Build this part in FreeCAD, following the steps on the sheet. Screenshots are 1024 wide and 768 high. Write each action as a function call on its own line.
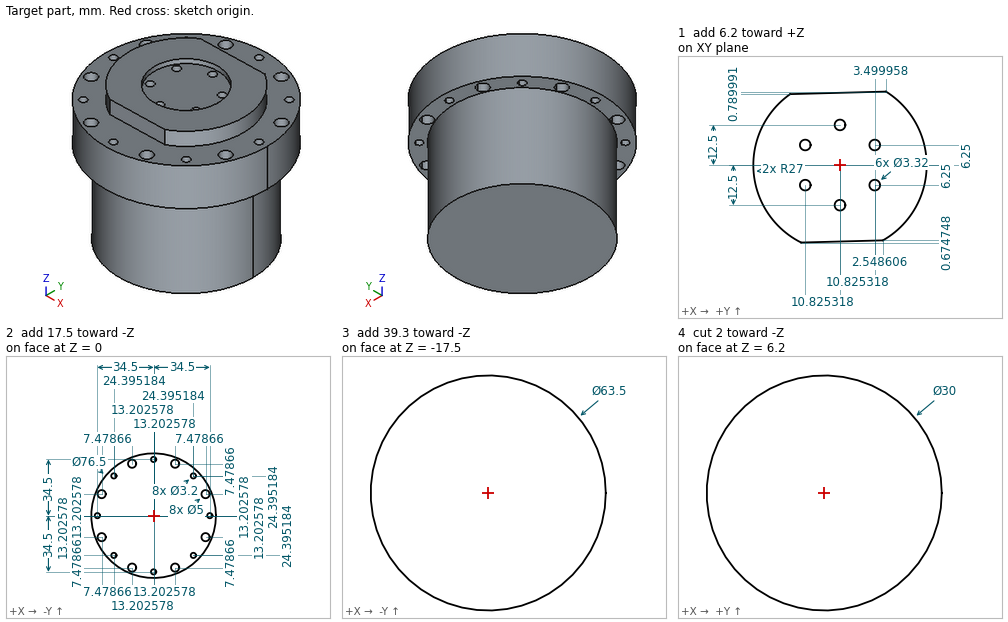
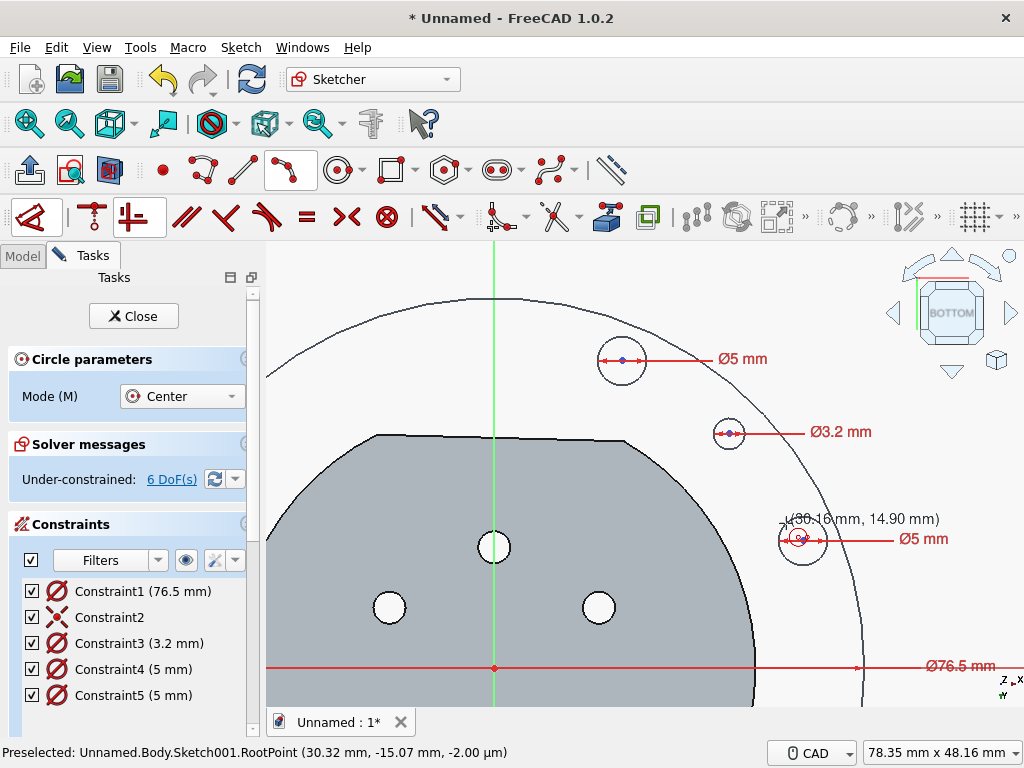
scroll(494, 334, up, 2)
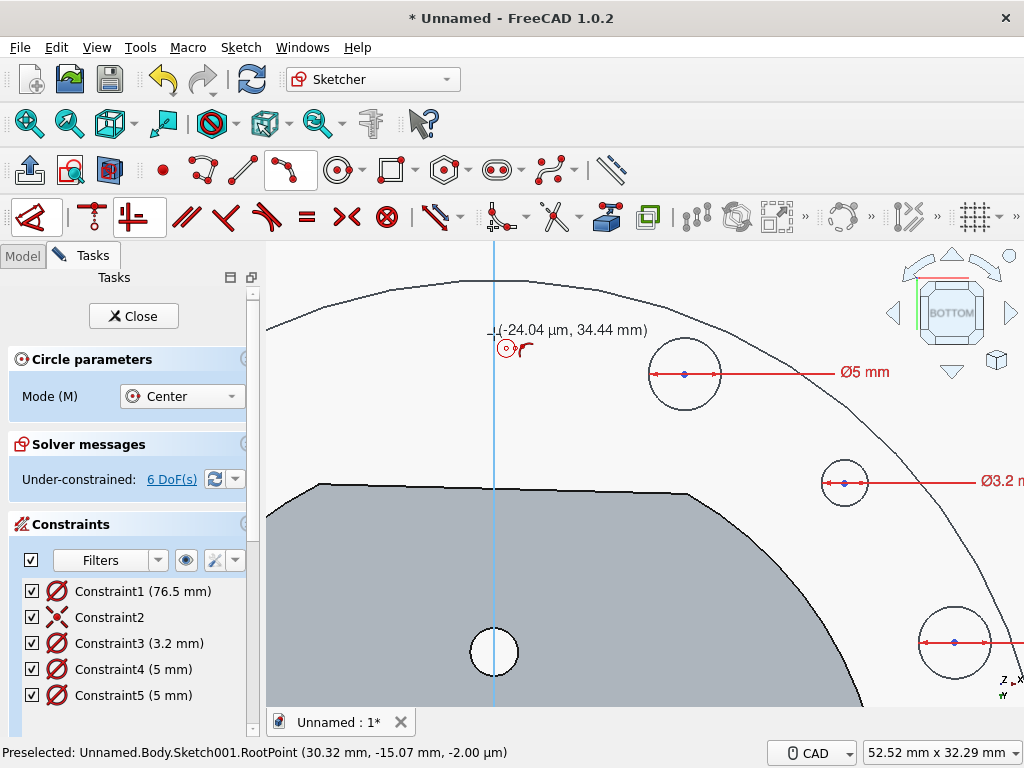
scroll(603, 357, down, 7)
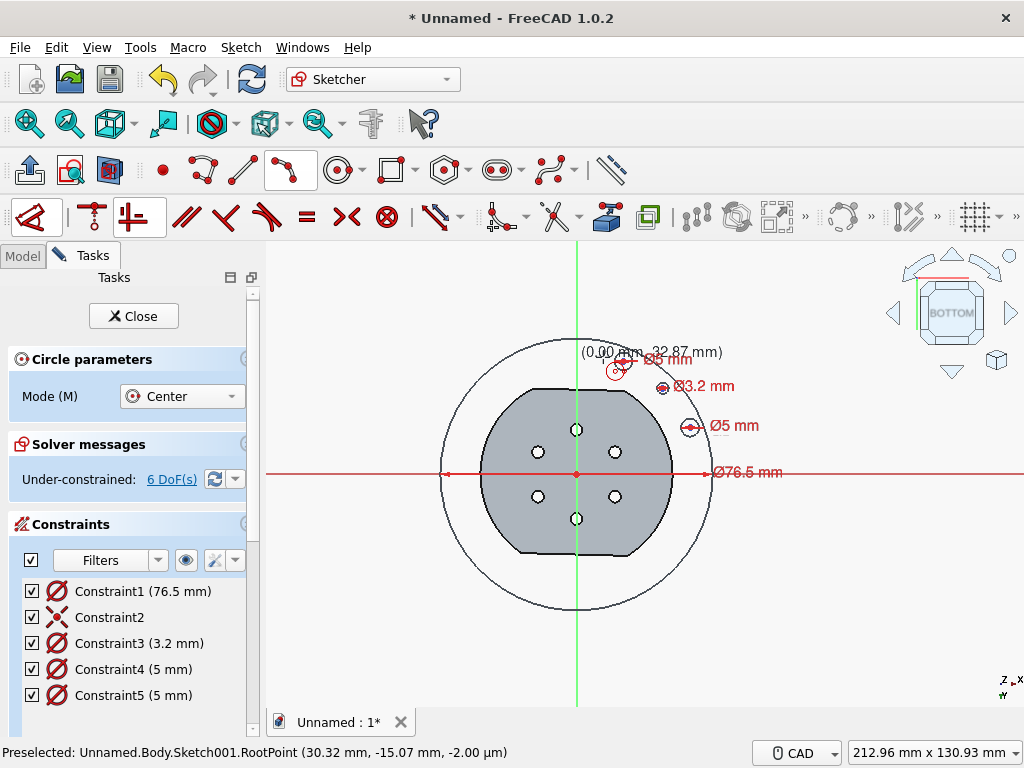
click(577, 352)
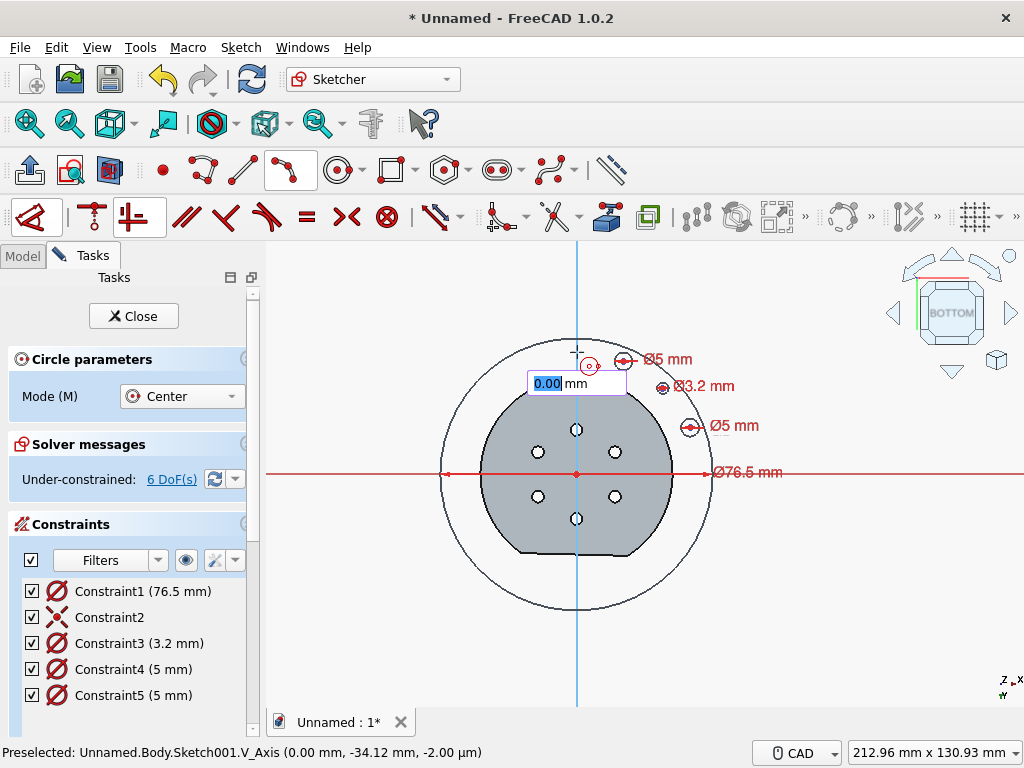
scroll(582, 350, up, 6)
move(581, 348)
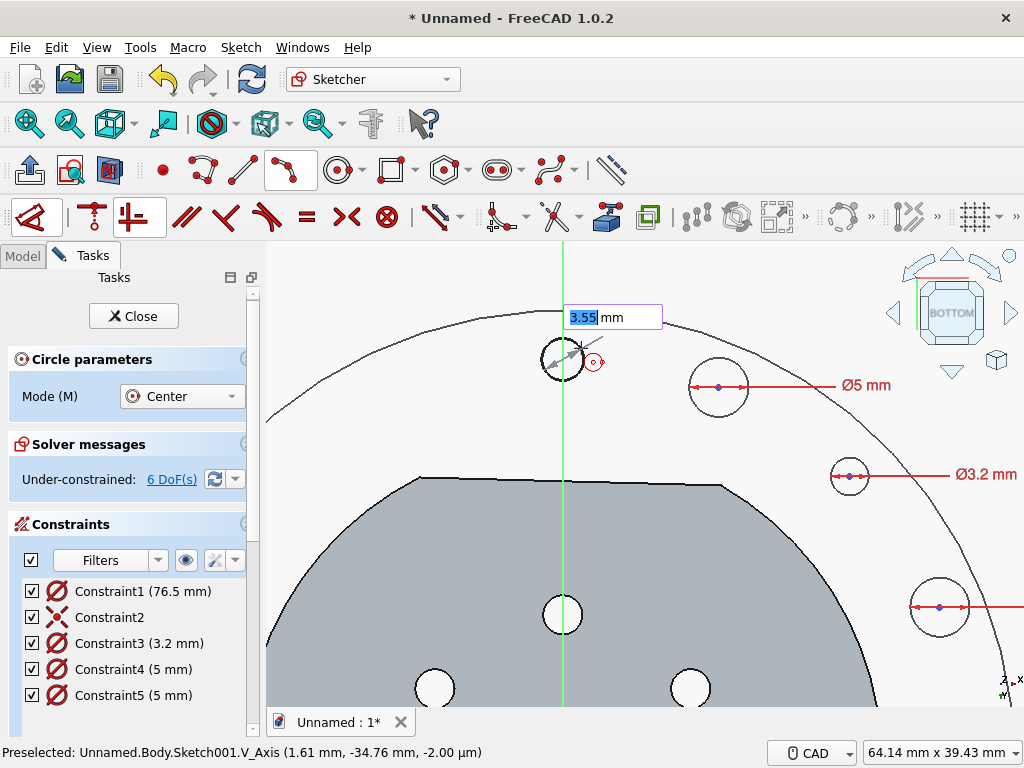
text(3.2)
key(Return)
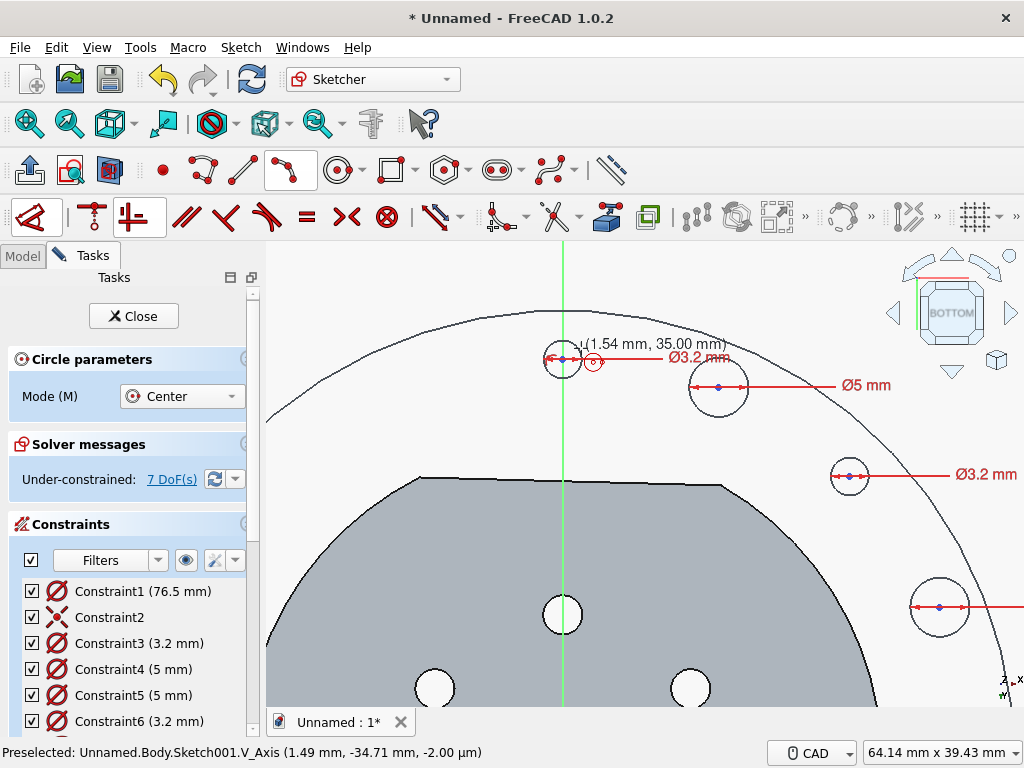
click(407, 386)
move(428, 365)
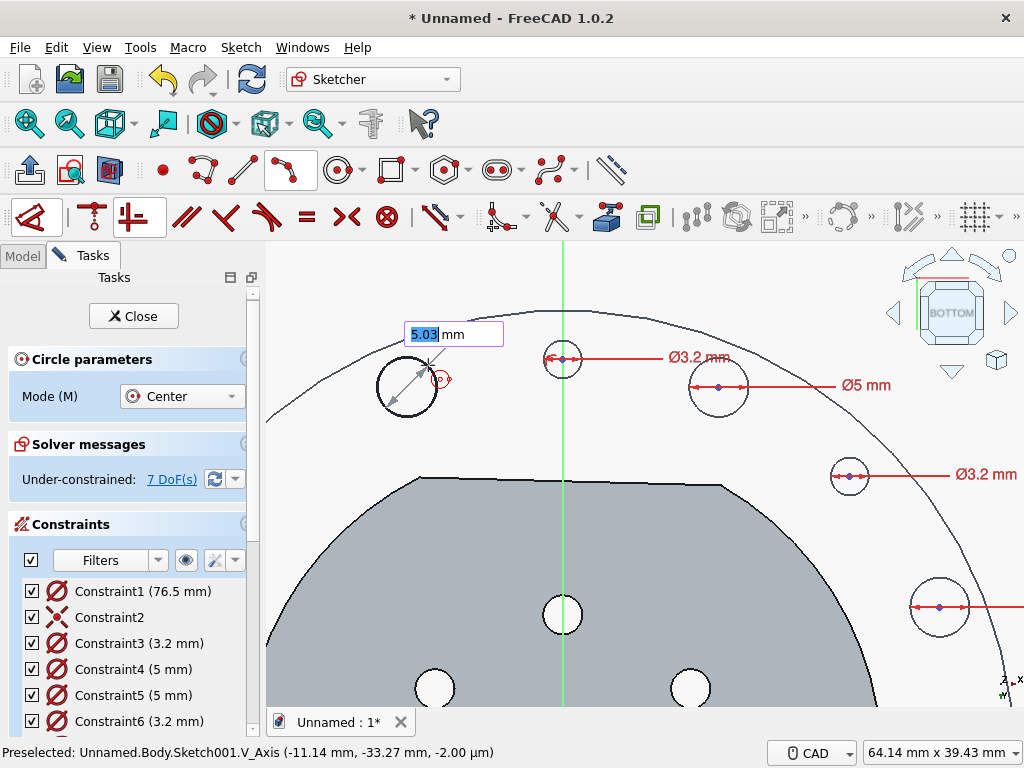
text(5)
key(Return)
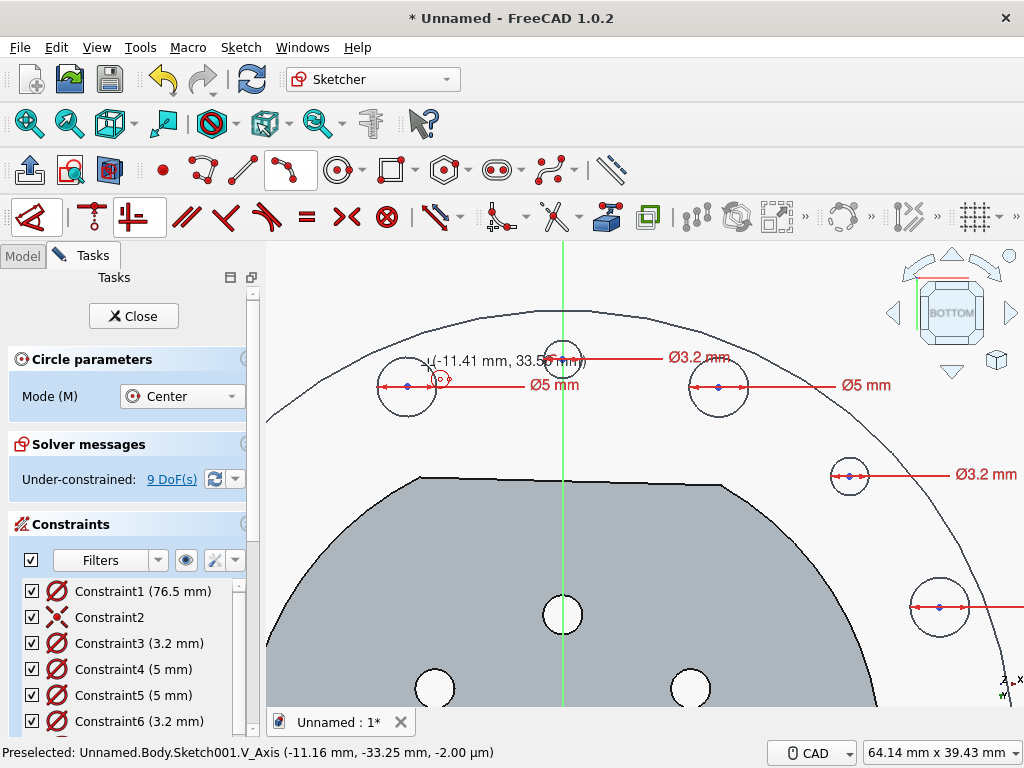
scroll(582, 350, down, 6)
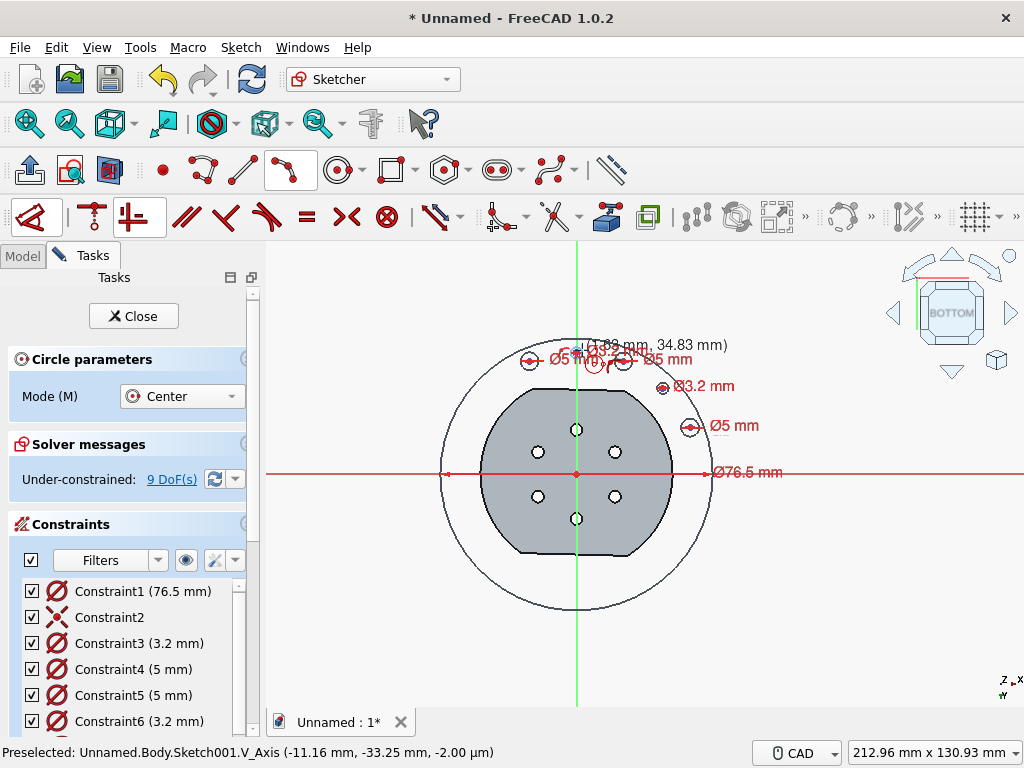
scroll(490, 388, up, 7)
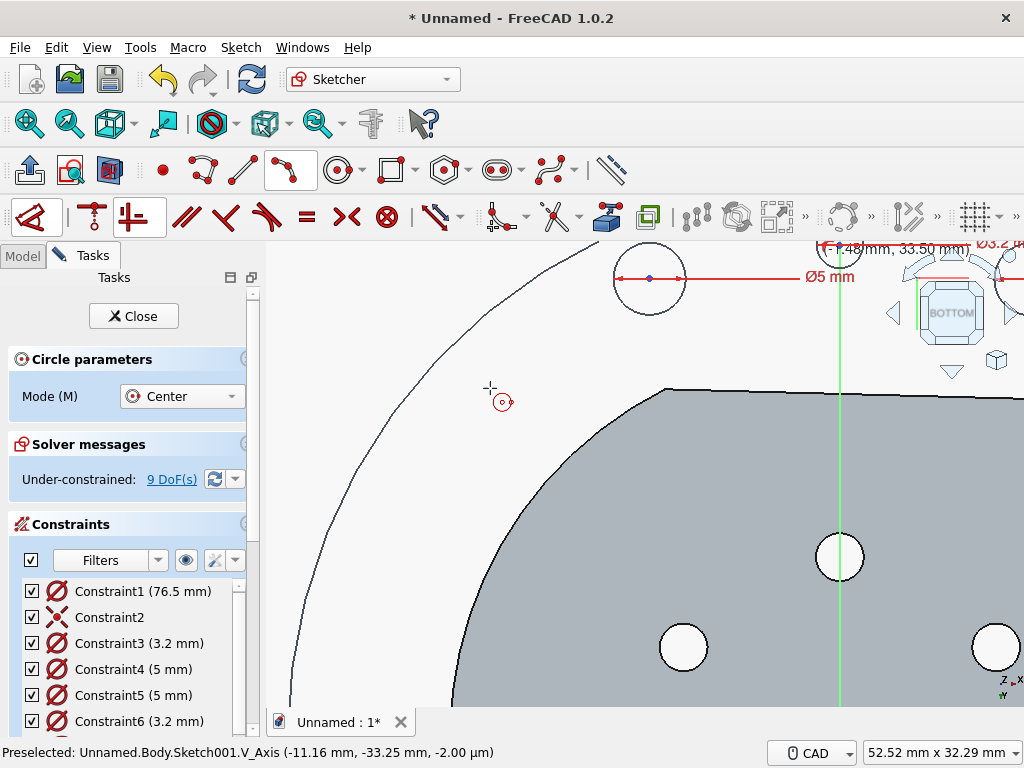
scroll(490, 388, down, 7)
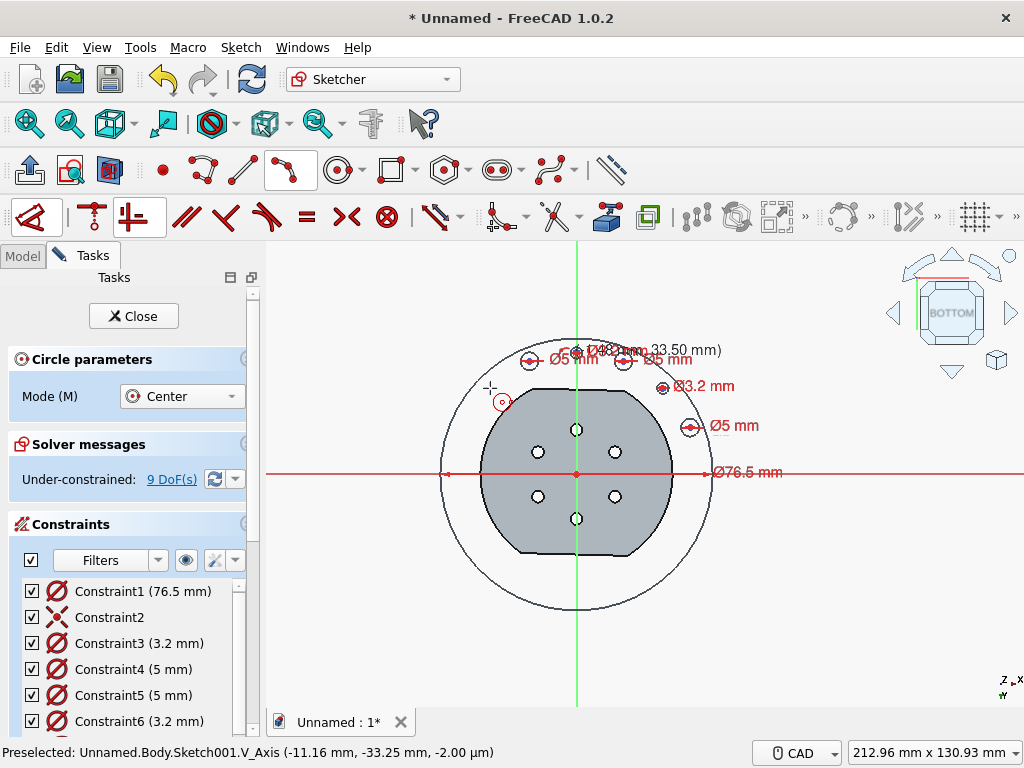
click(490, 388)
move(494, 392)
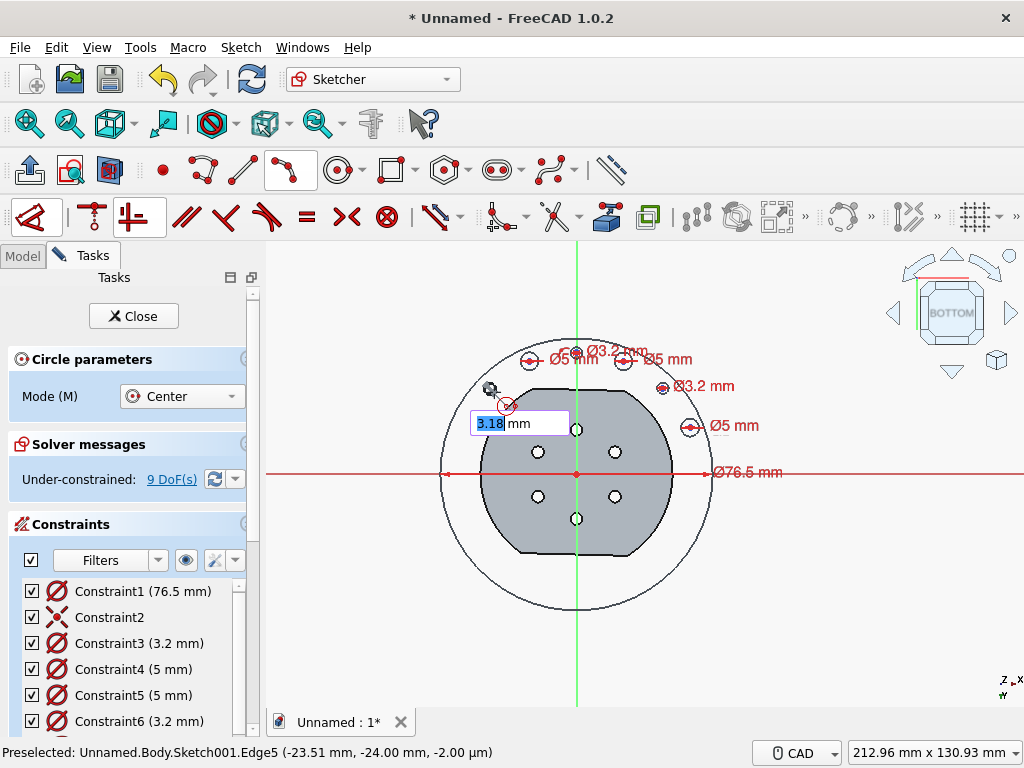
text(3.2)
key(Return)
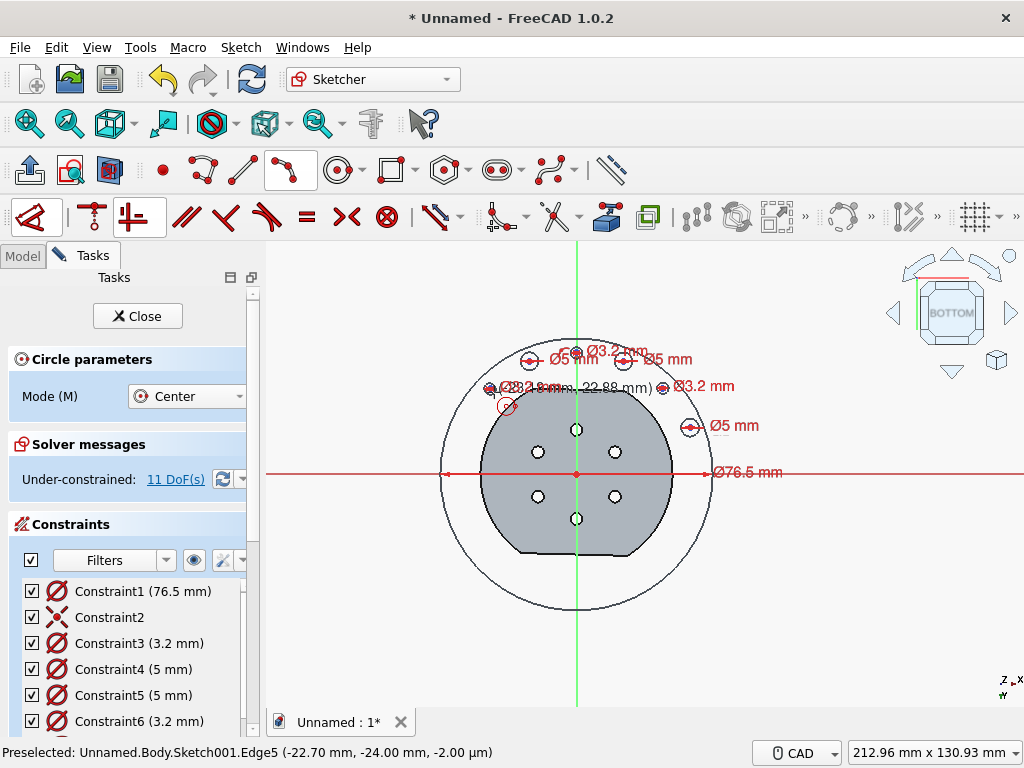
scroll(463, 427, up, 5)